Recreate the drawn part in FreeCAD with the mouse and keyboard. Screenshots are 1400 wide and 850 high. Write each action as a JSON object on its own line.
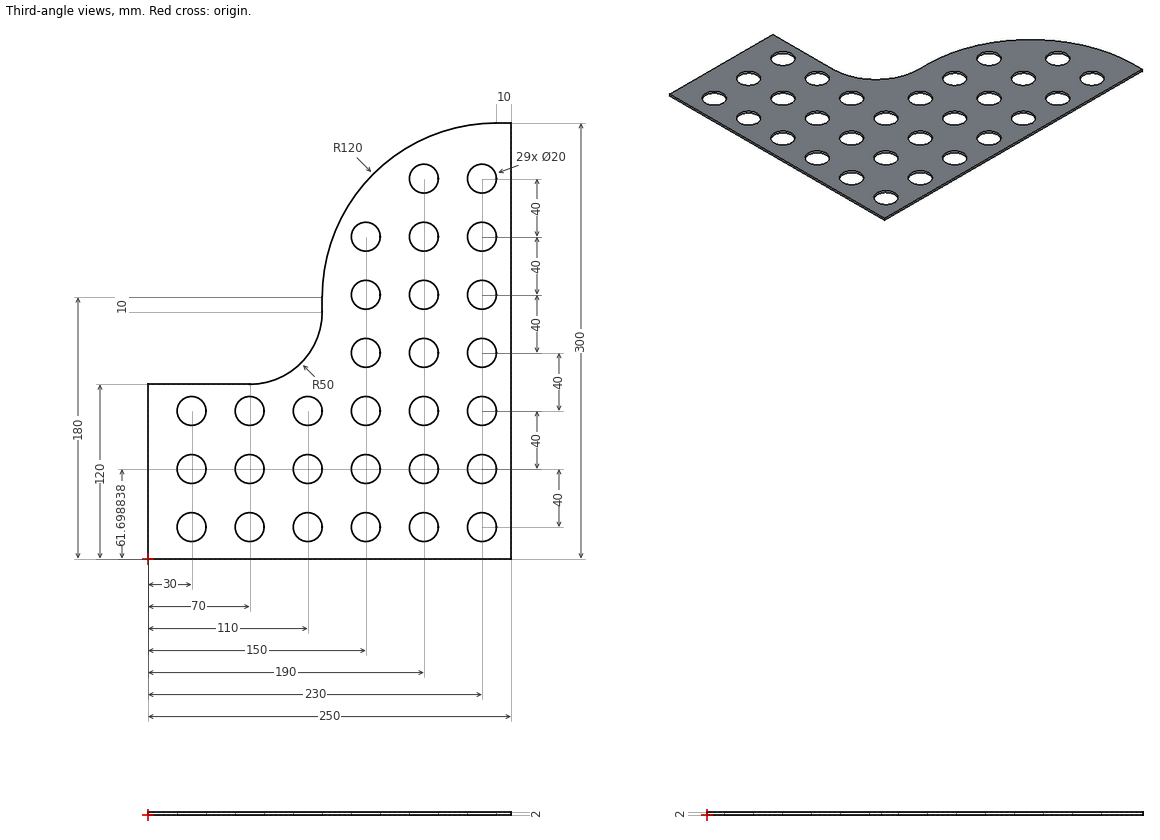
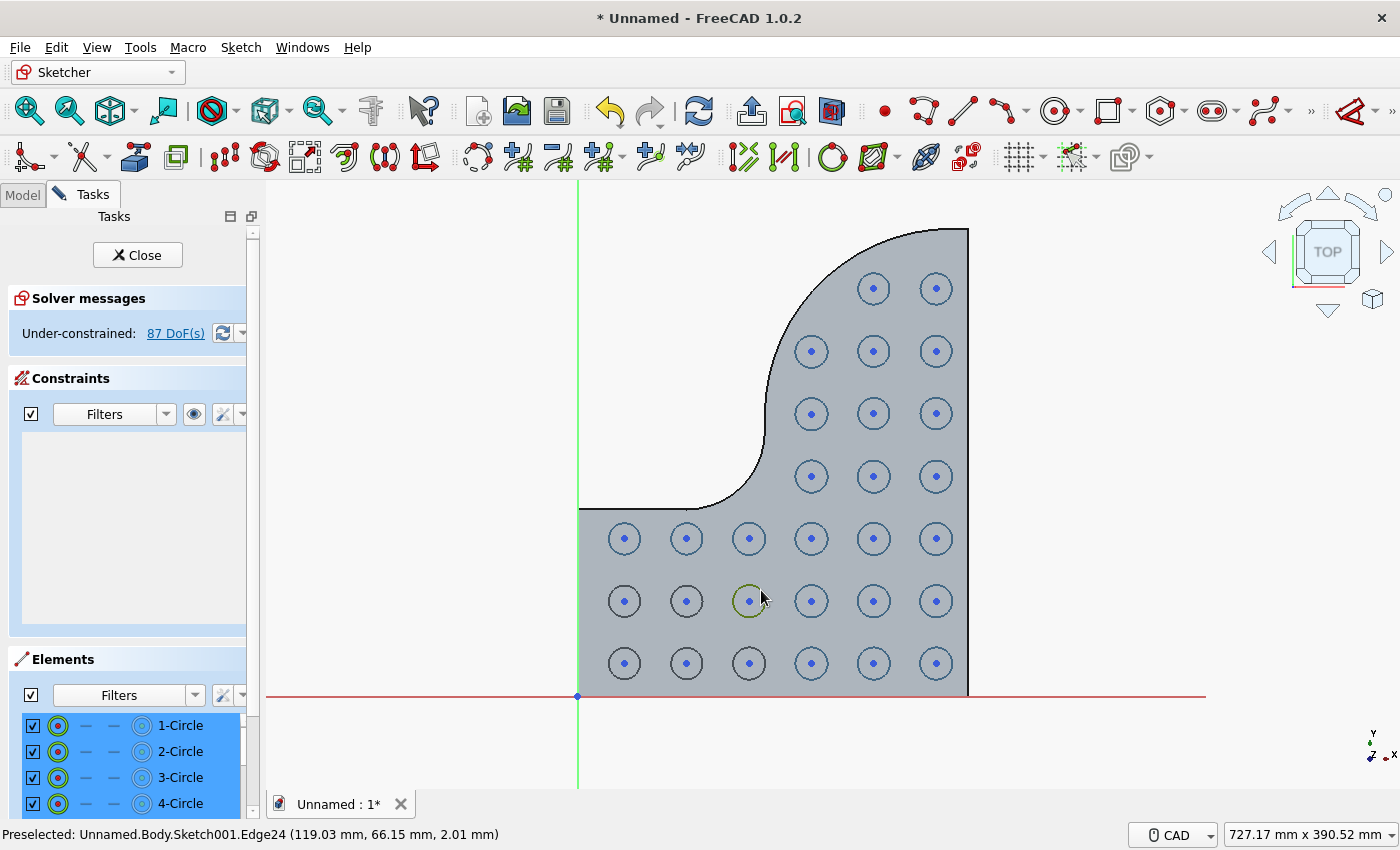
{"action": "left_click", "coordinate": [698, 590]}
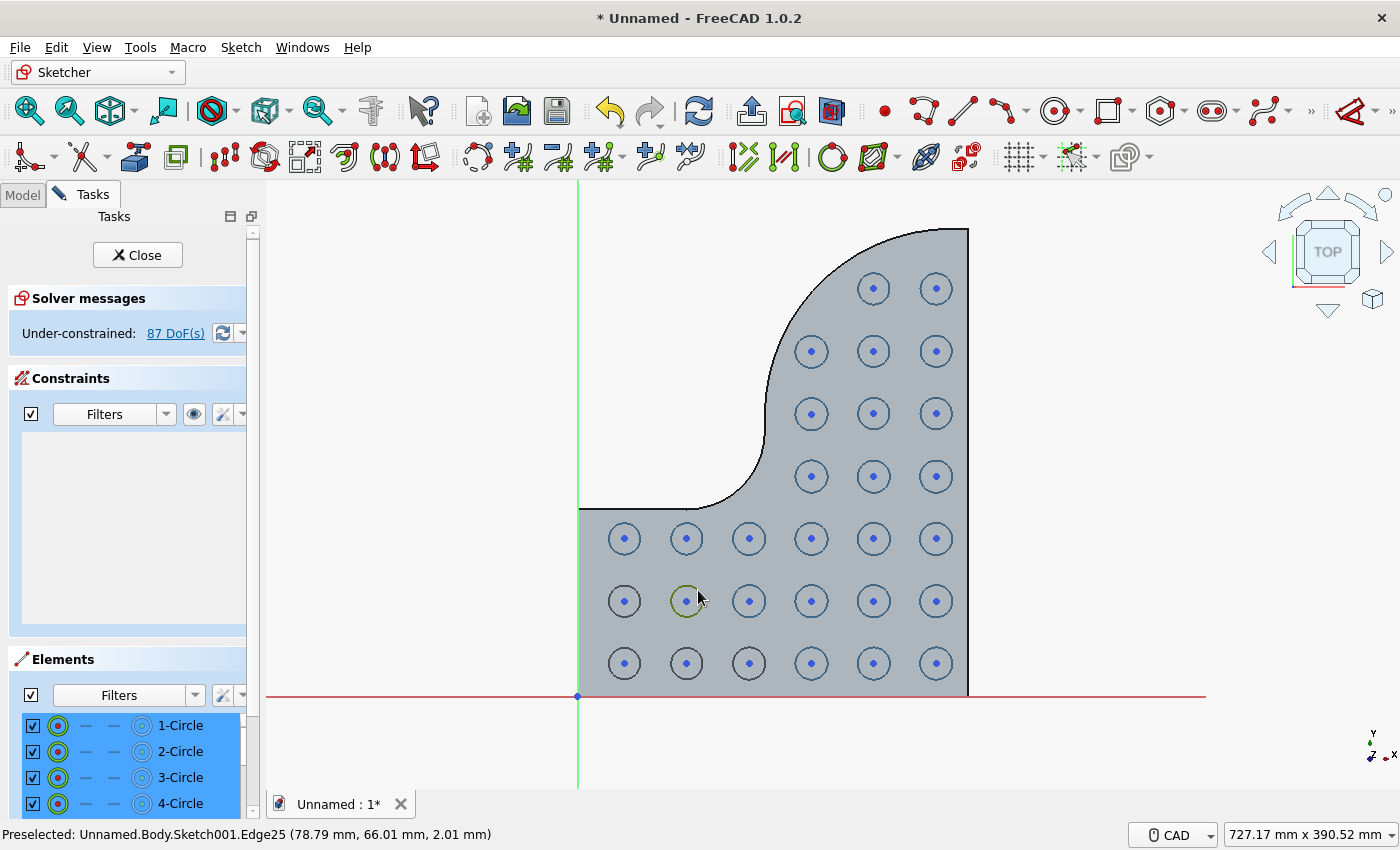
{"action": "left_click", "coordinate": [636, 590]}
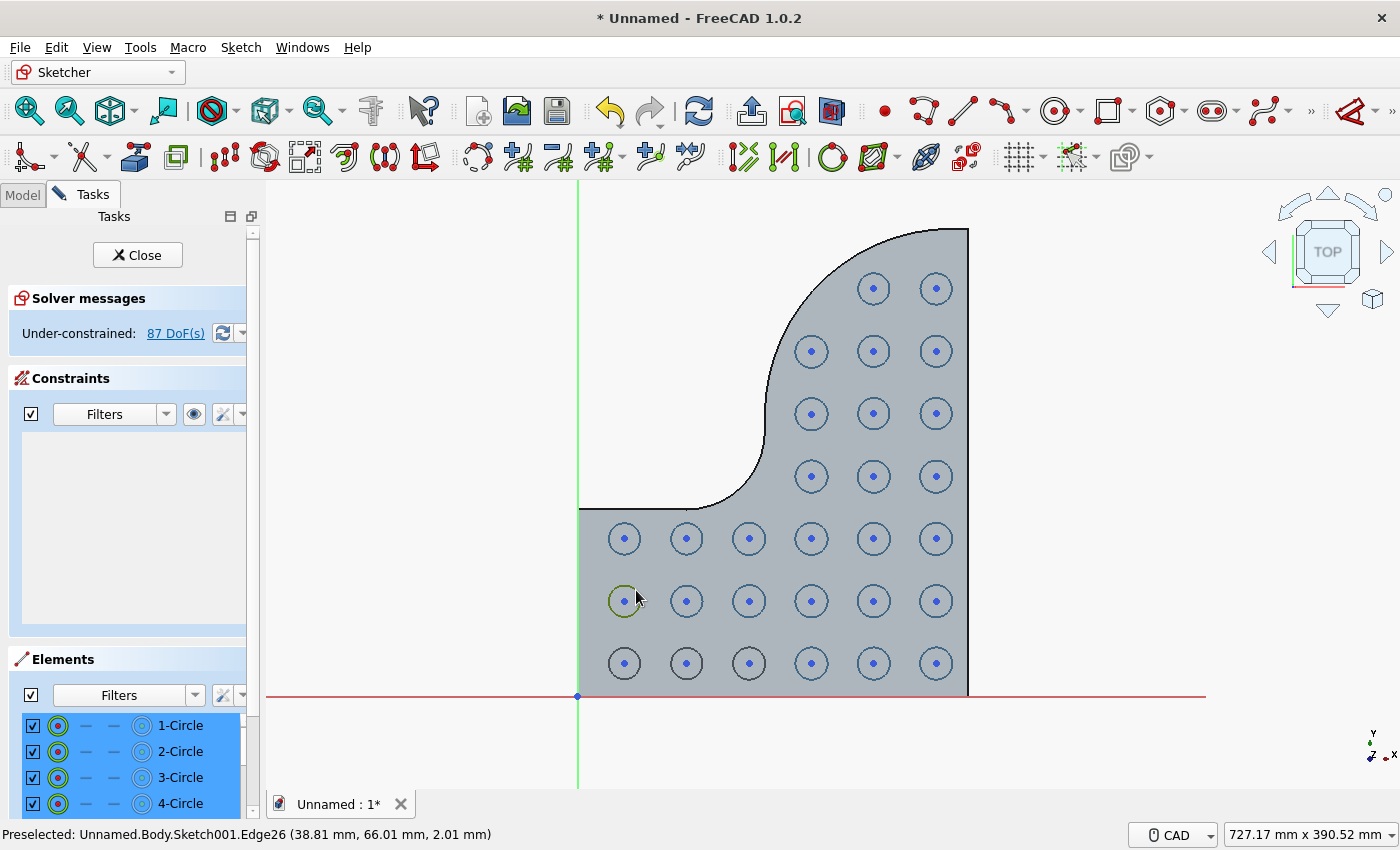
{"action": "left_click", "coordinate": [761, 652]}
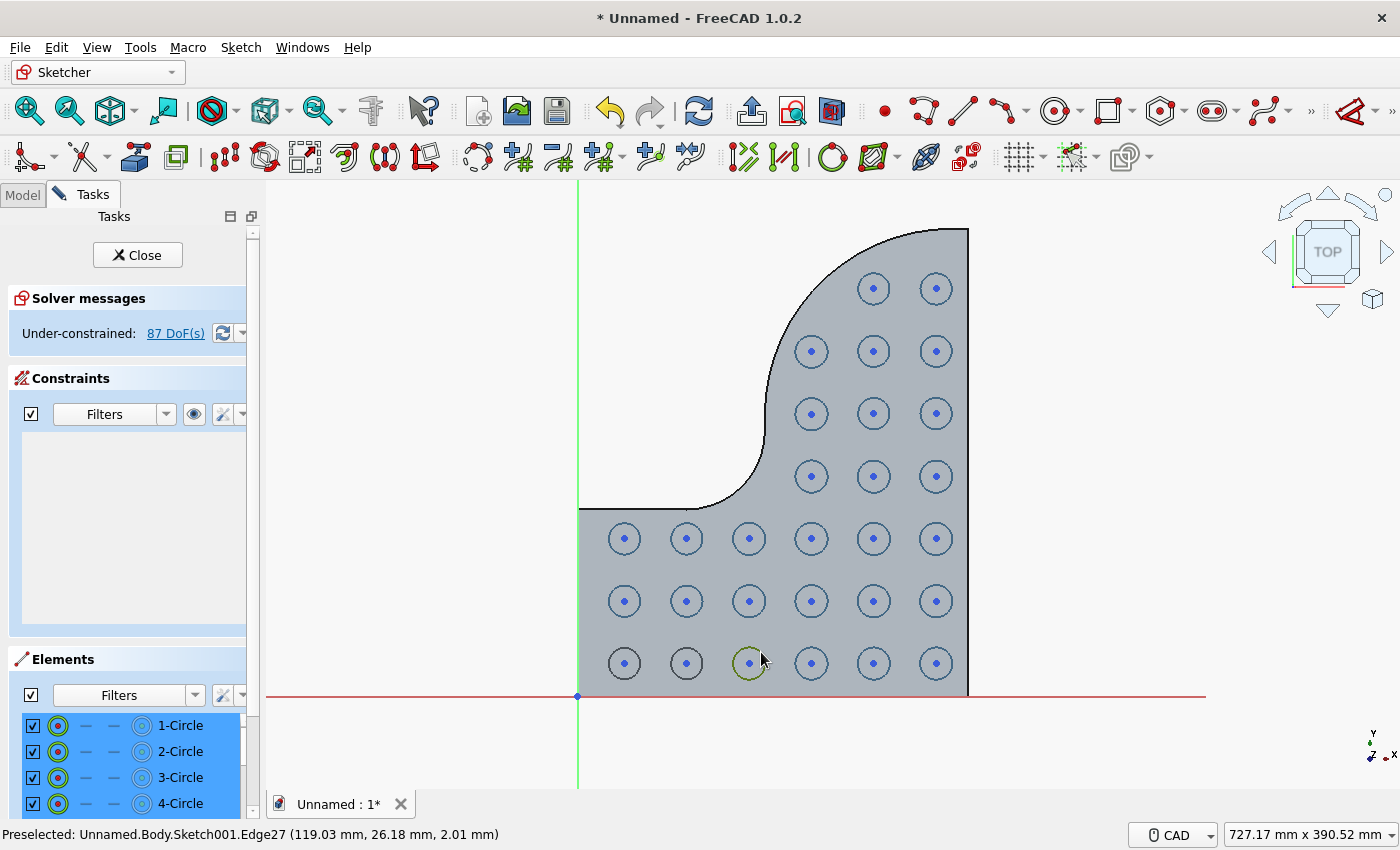
{"action": "left_click", "coordinate": [698, 652]}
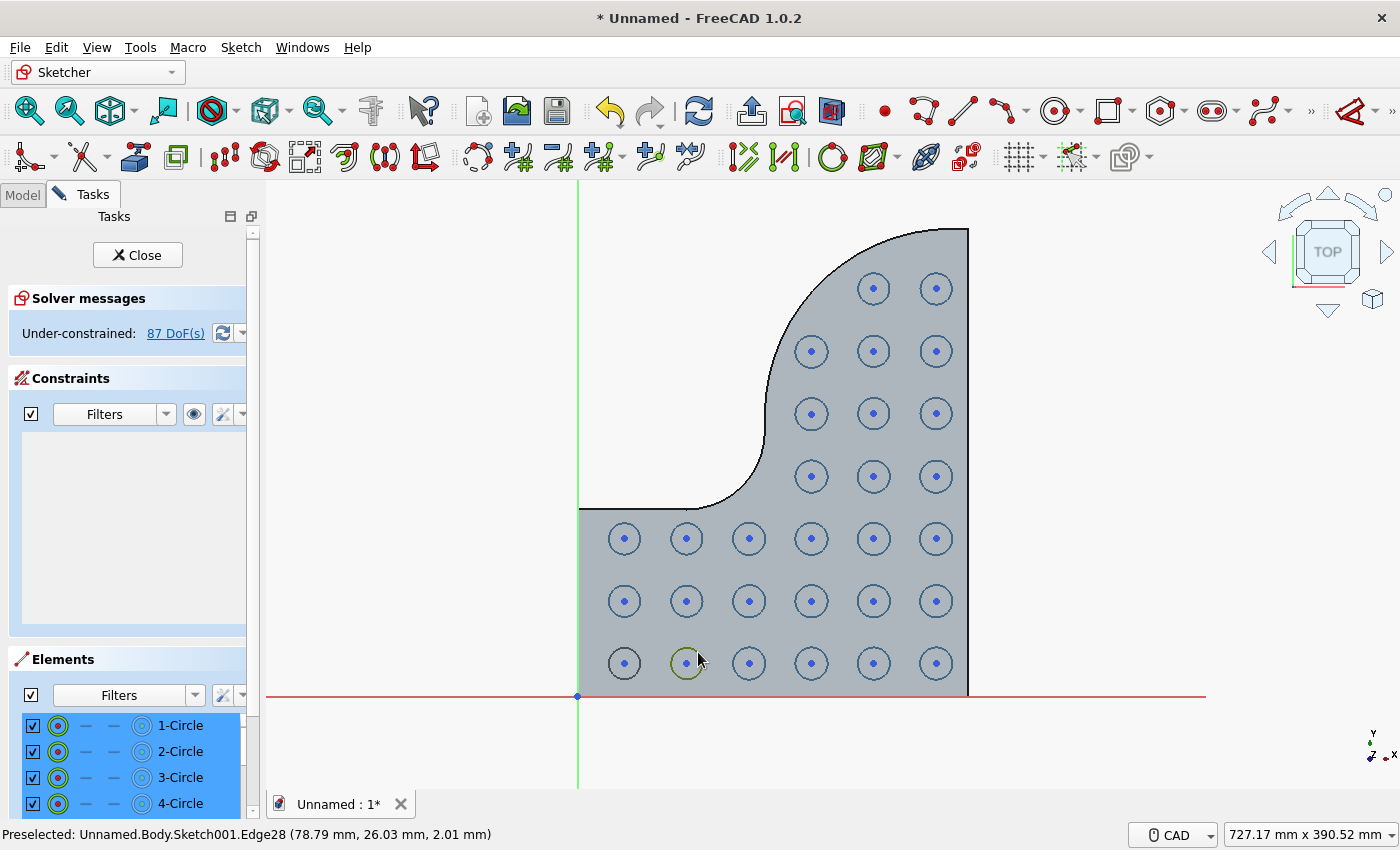
{"action": "left_click", "coordinate": [636, 652]}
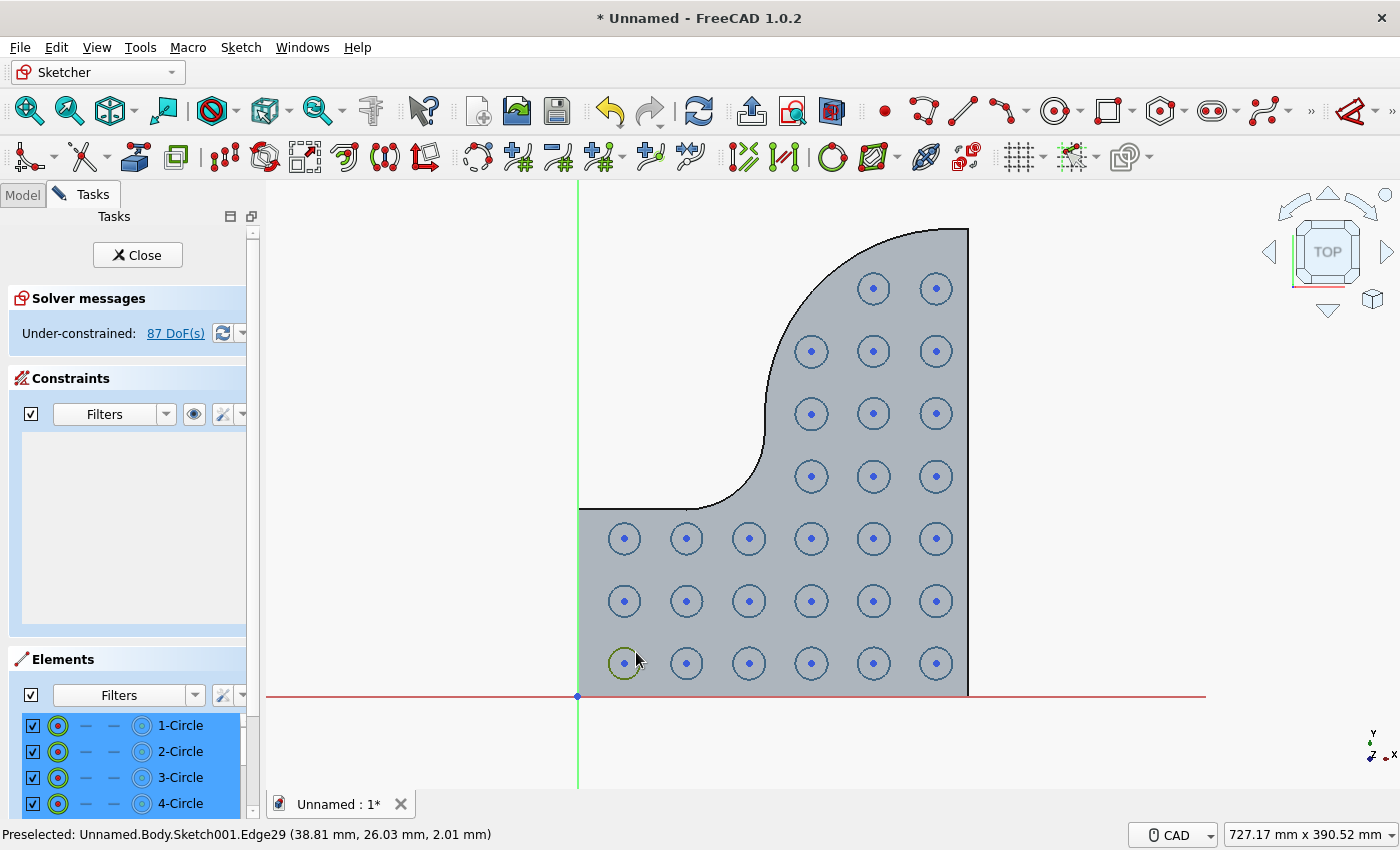
{"action": "key", "text": "e"}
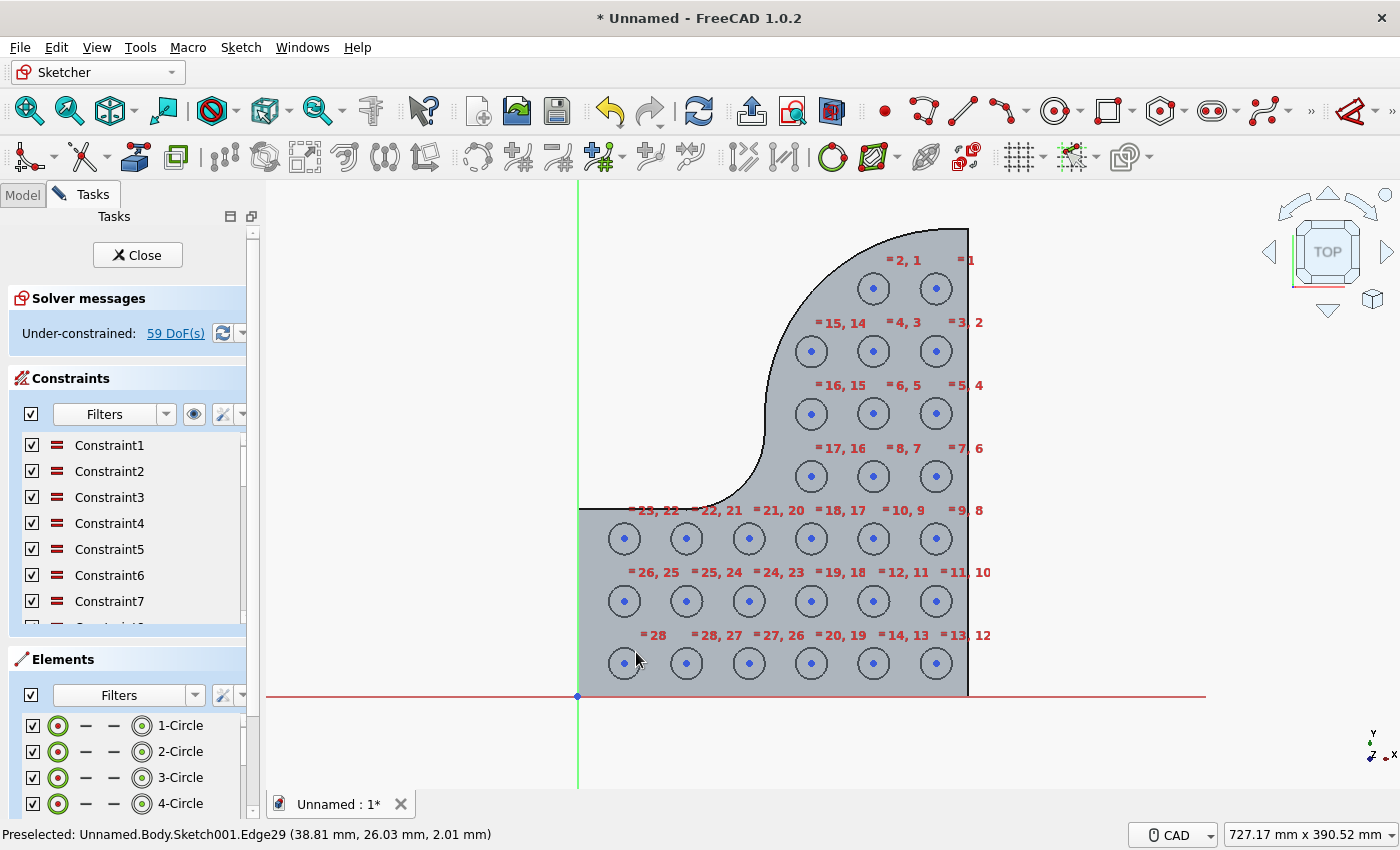
{"action": "left_click", "coordinate": [1350, 112]}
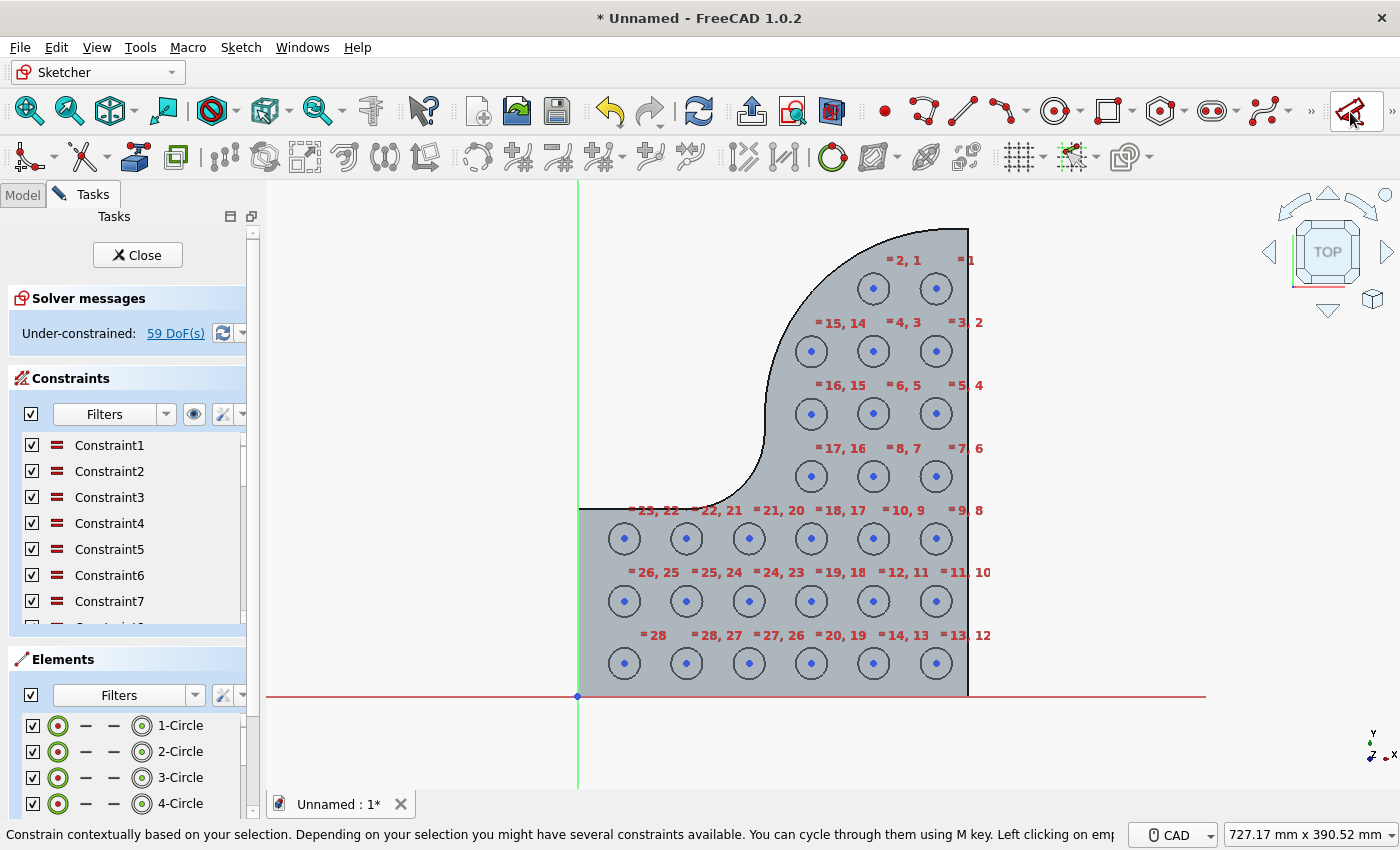
{"action": "scroll", "coordinate": [947, 278], "scroll_direction": "up", "scroll_amount": 2}